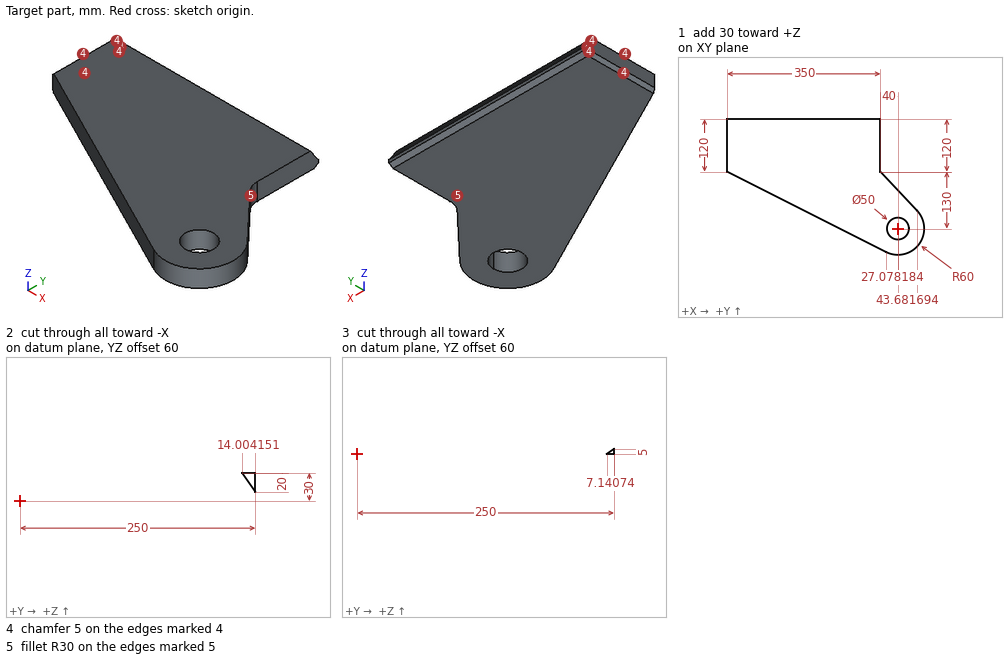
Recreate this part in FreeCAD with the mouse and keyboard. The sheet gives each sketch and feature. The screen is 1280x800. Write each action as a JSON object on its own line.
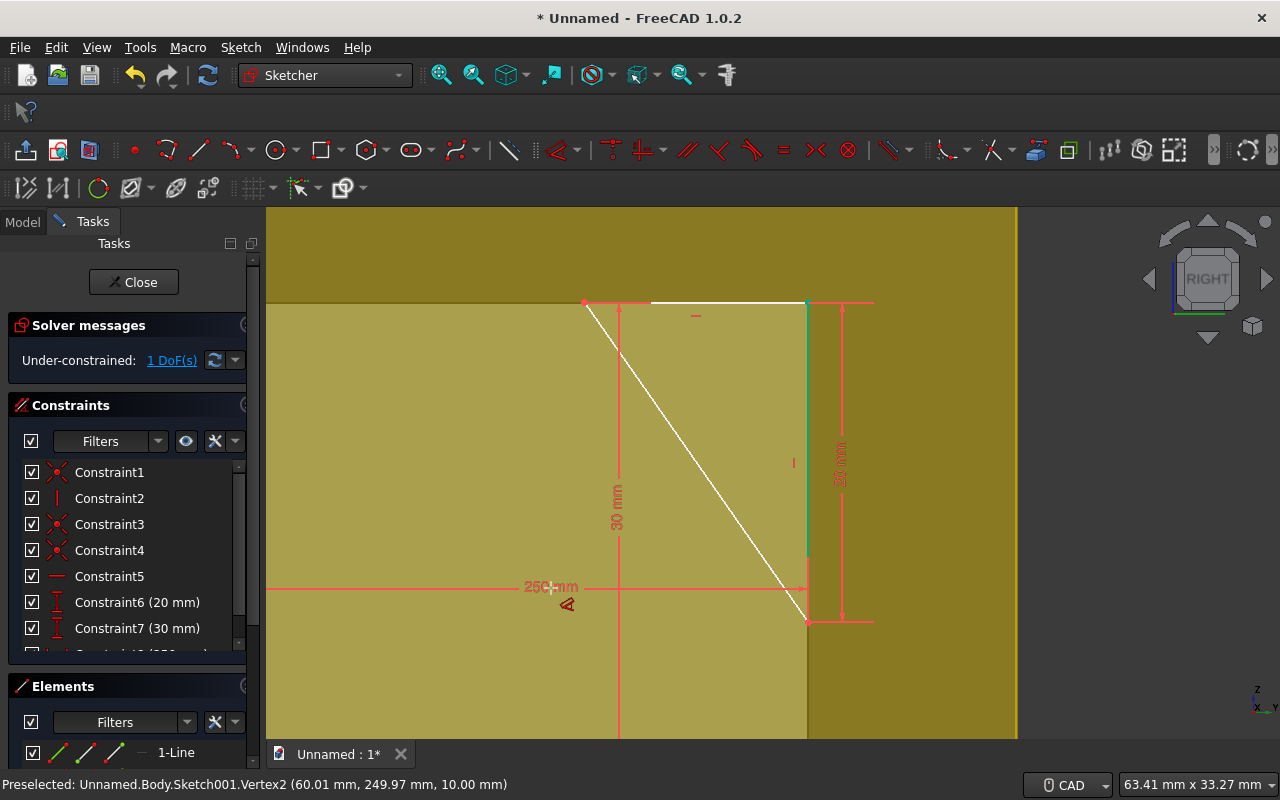
{"action": "left_click", "coordinate": [741, 303]}
{"action": "left_click", "coordinate": [696, 269]}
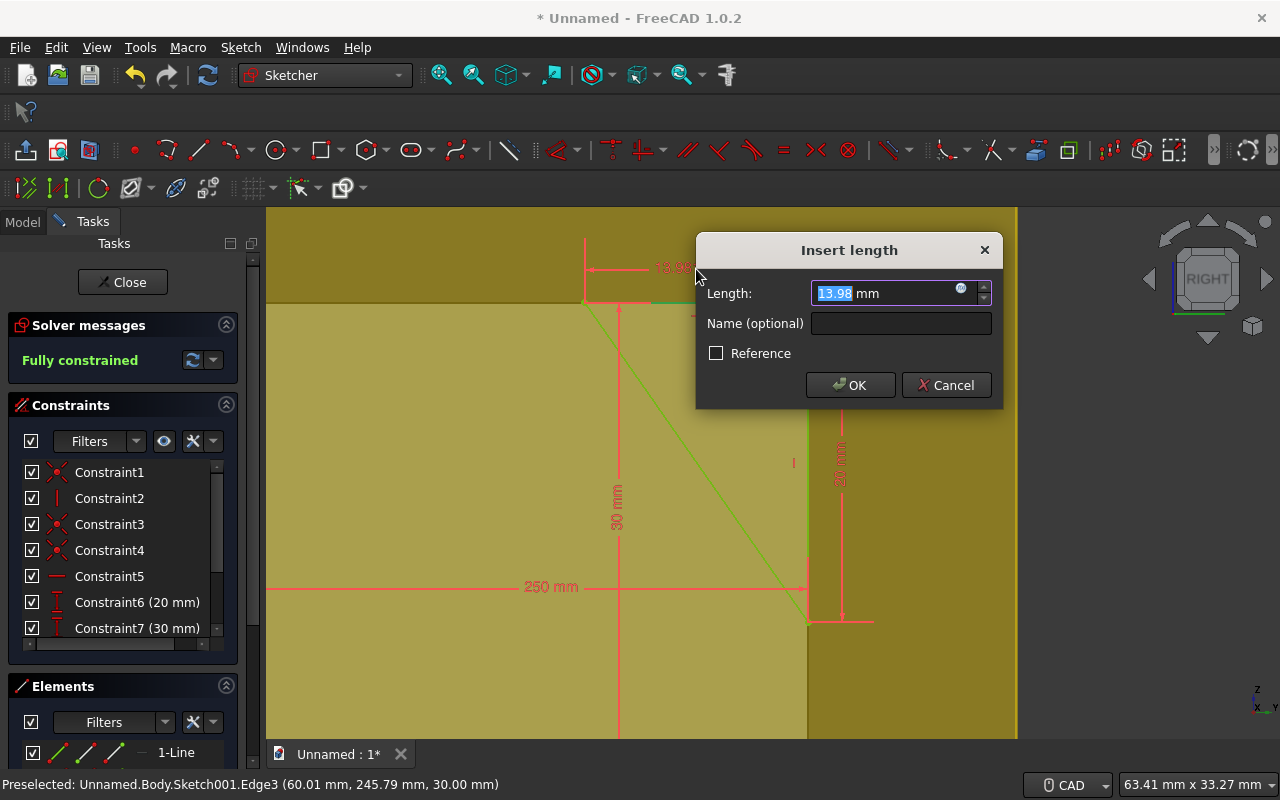
{"action": "type", "text": "14.004151"}
{"action": "key", "text": "Return"}
{"action": "key", "text": "Escape"}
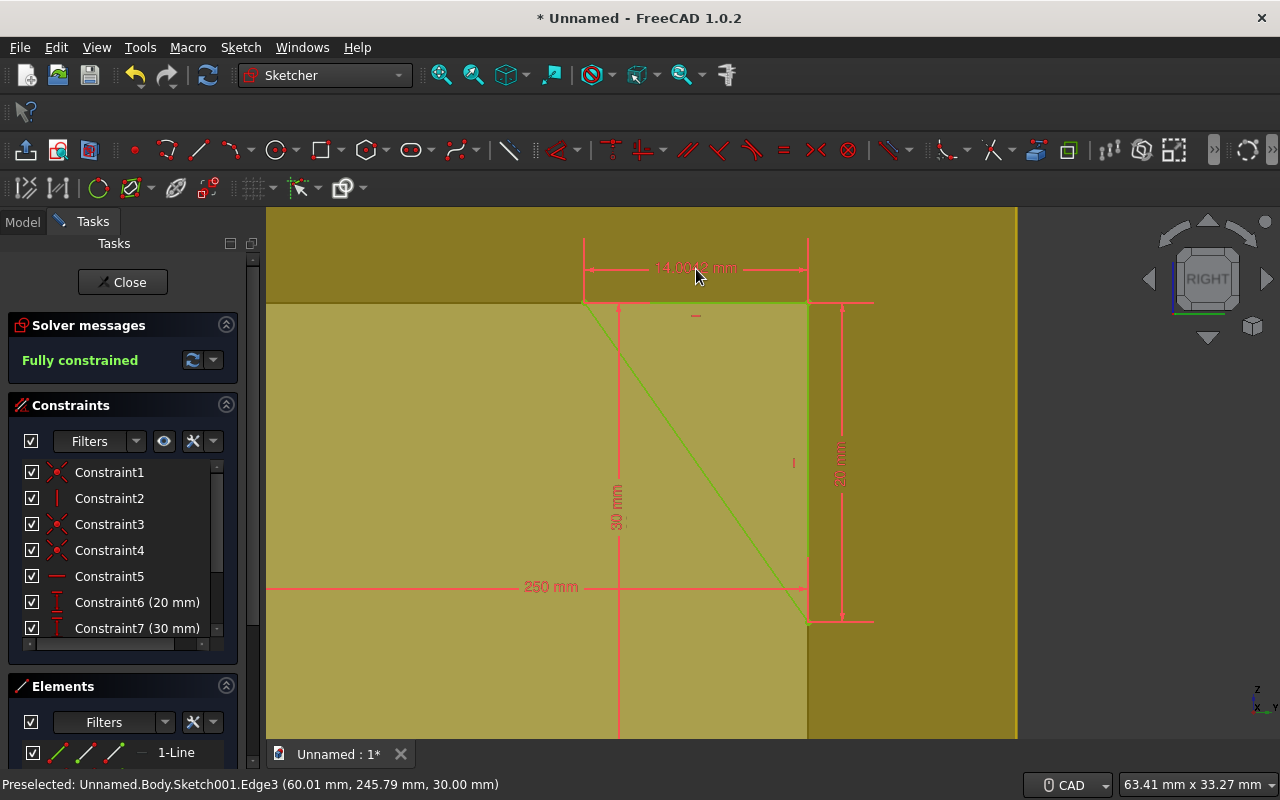
{"action": "left_click", "coordinate": [123, 282]}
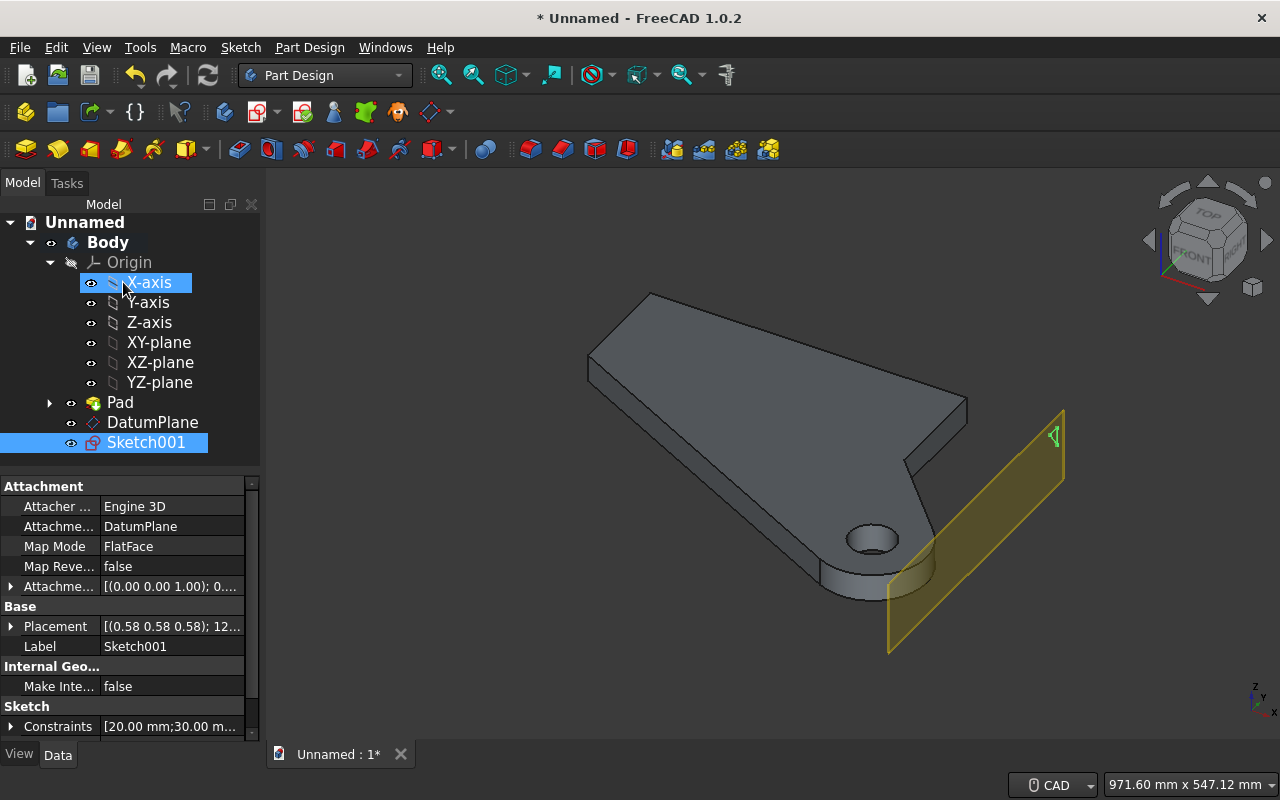
{"action": "left_click", "coordinate": [240, 150]}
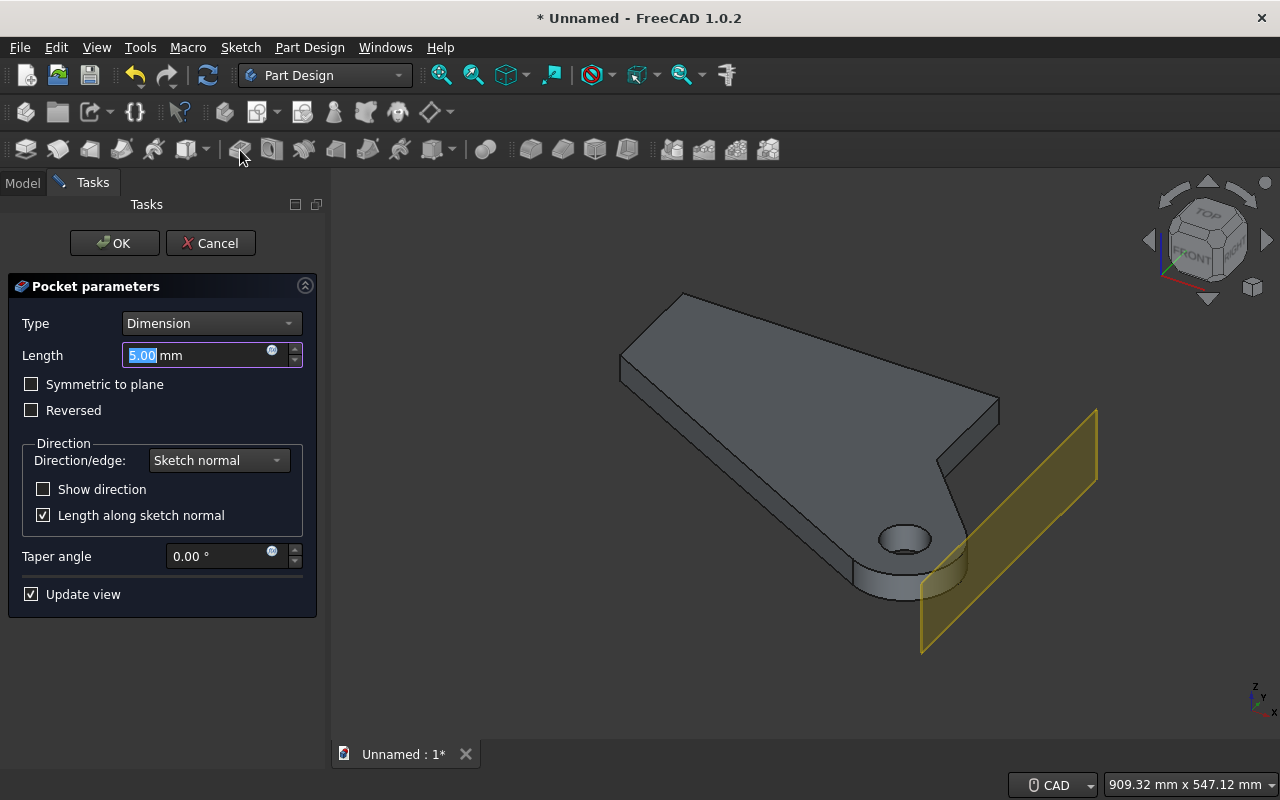
{"action": "left_click", "coordinate": [212, 324]}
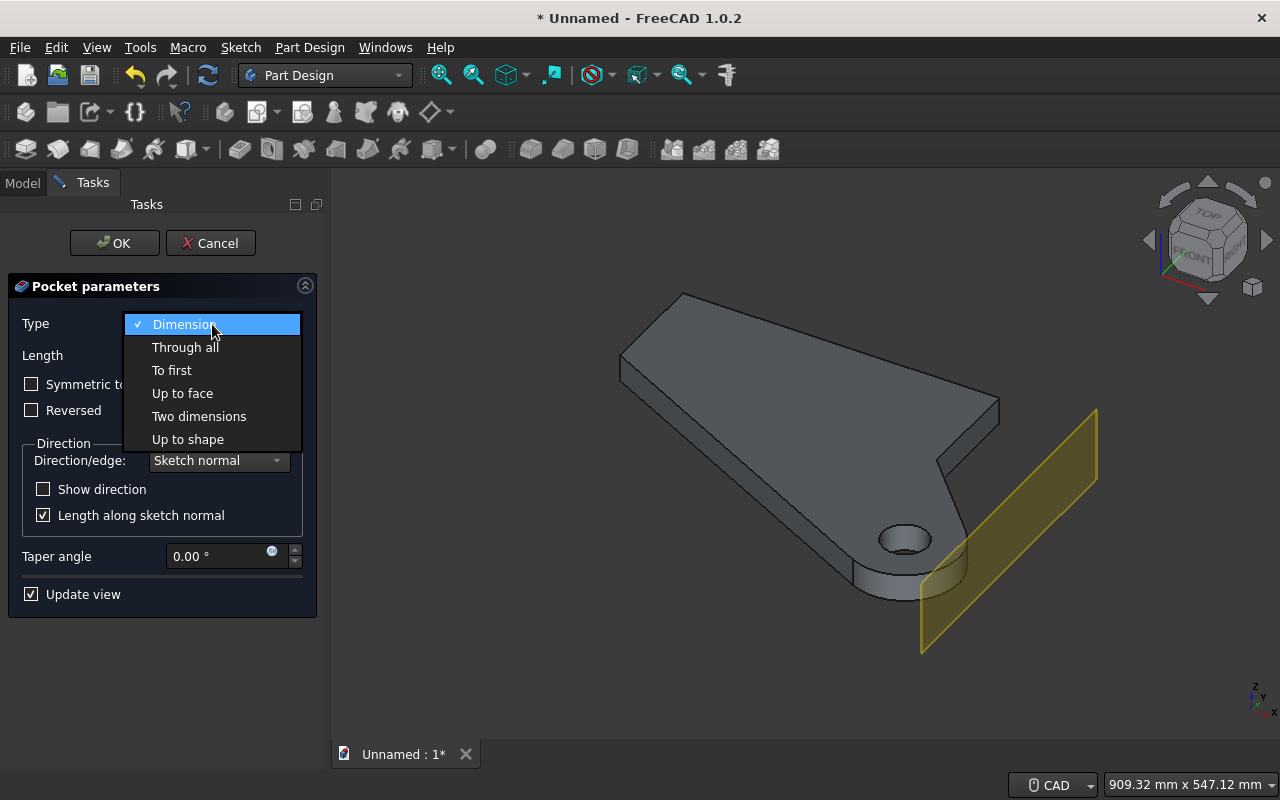
{"action": "left_click", "coordinate": [212, 348]}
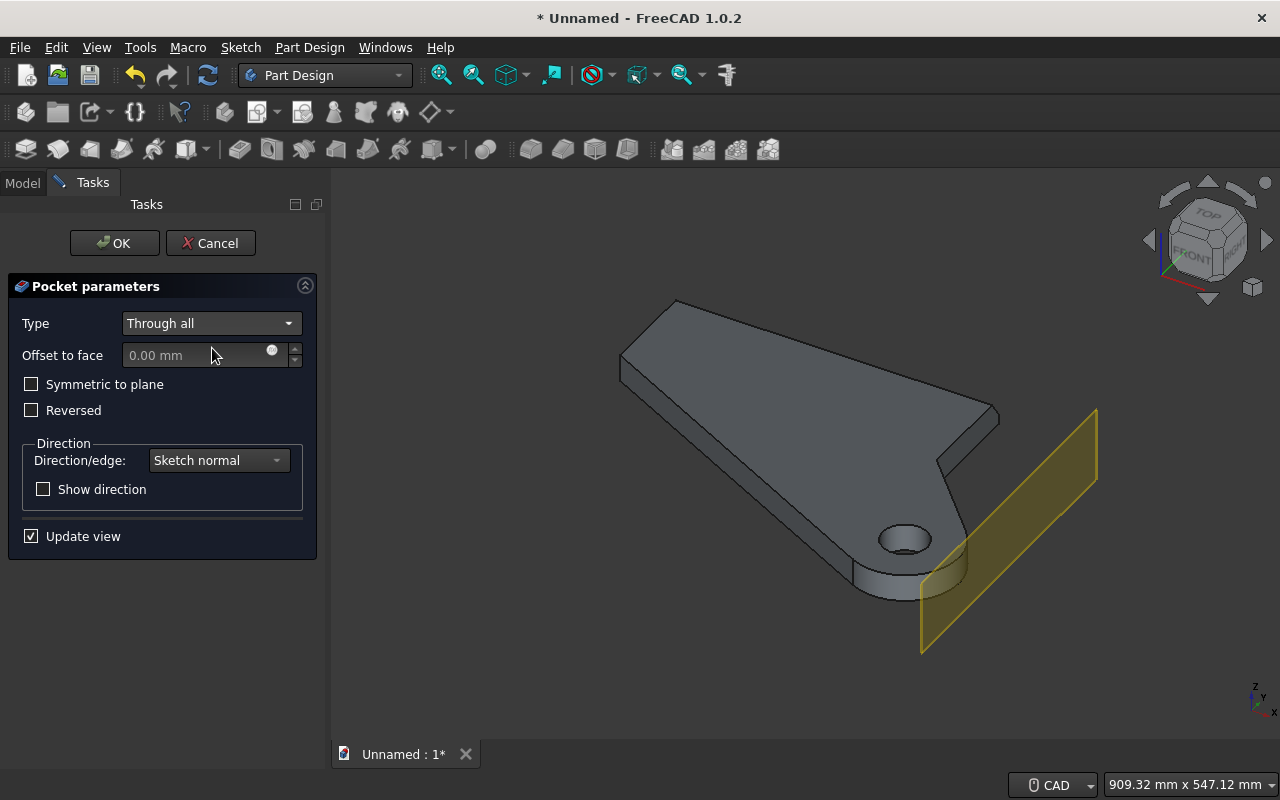
{"action": "left_click", "coordinate": [115, 243]}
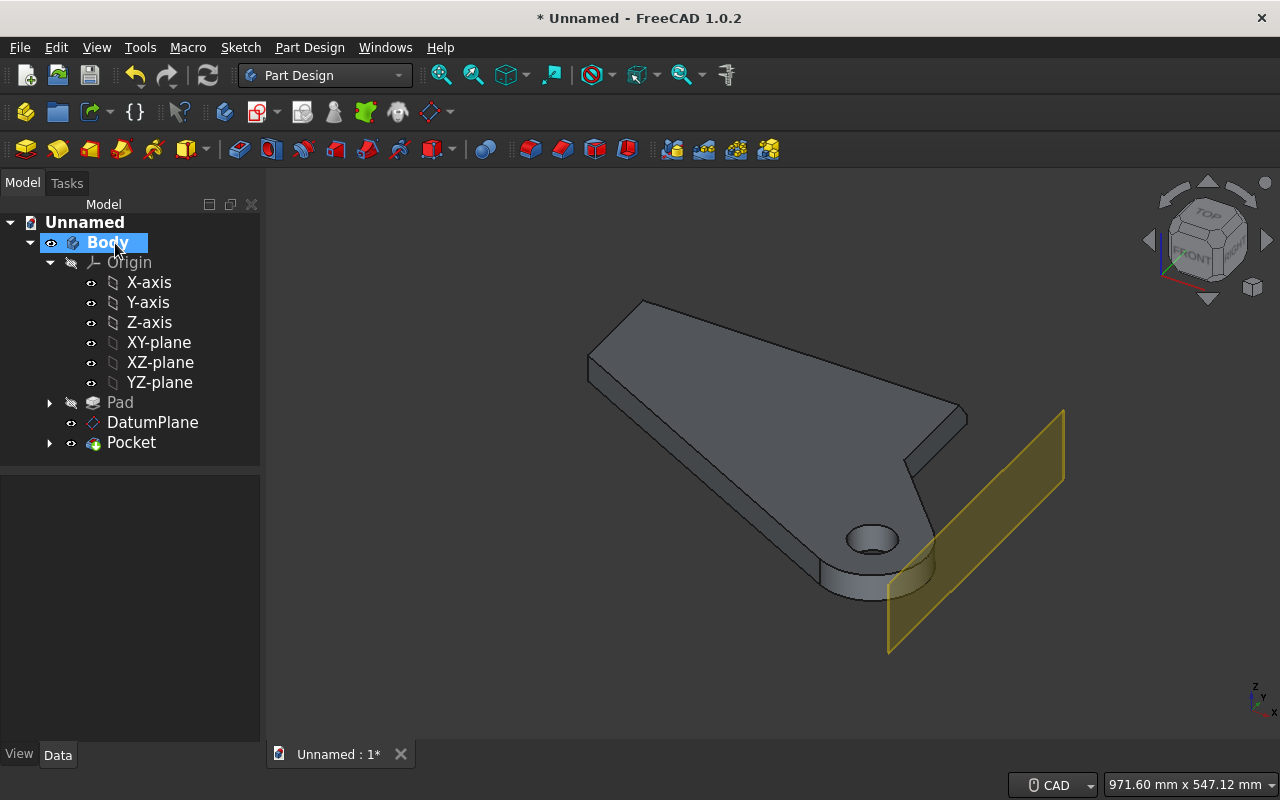
{"action": "left_click", "coordinate": [116, 423]}
{"action": "key", "text": "space"}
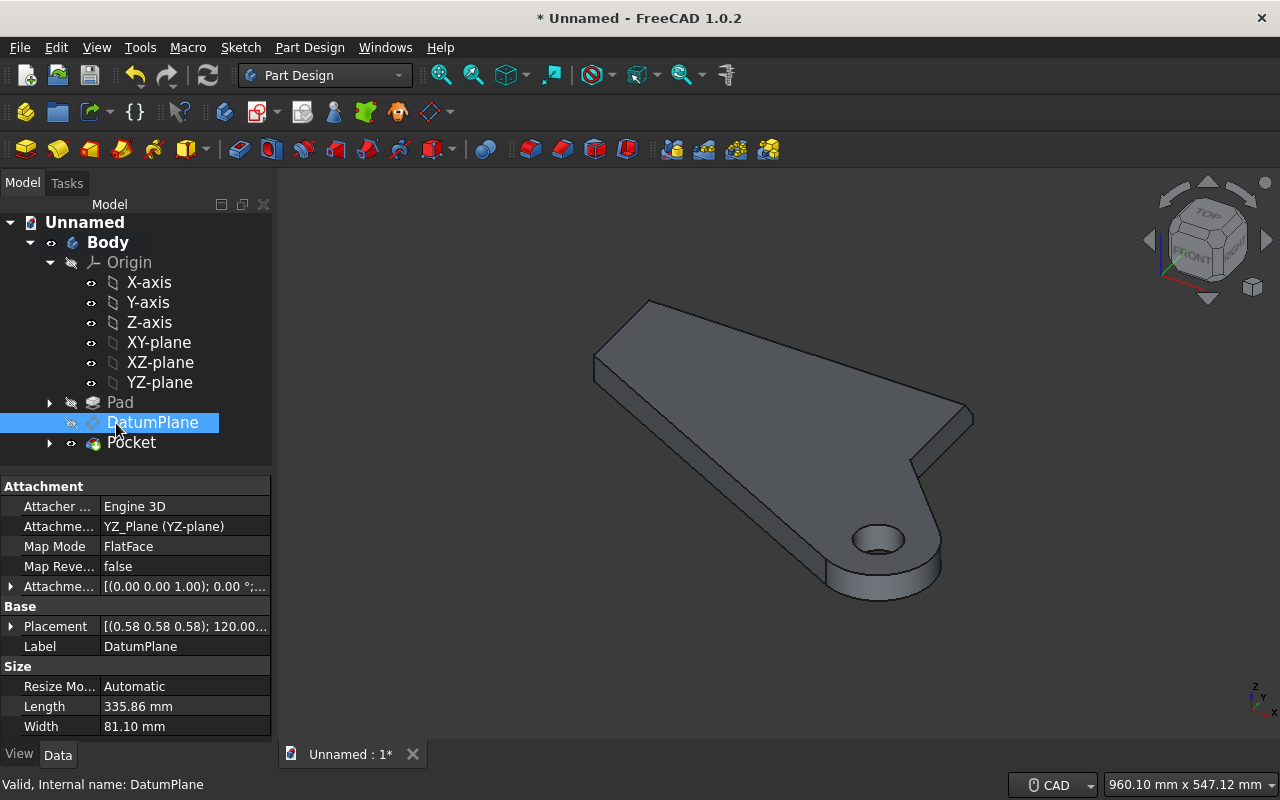
{"action": "left_click", "coordinate": [136, 383]}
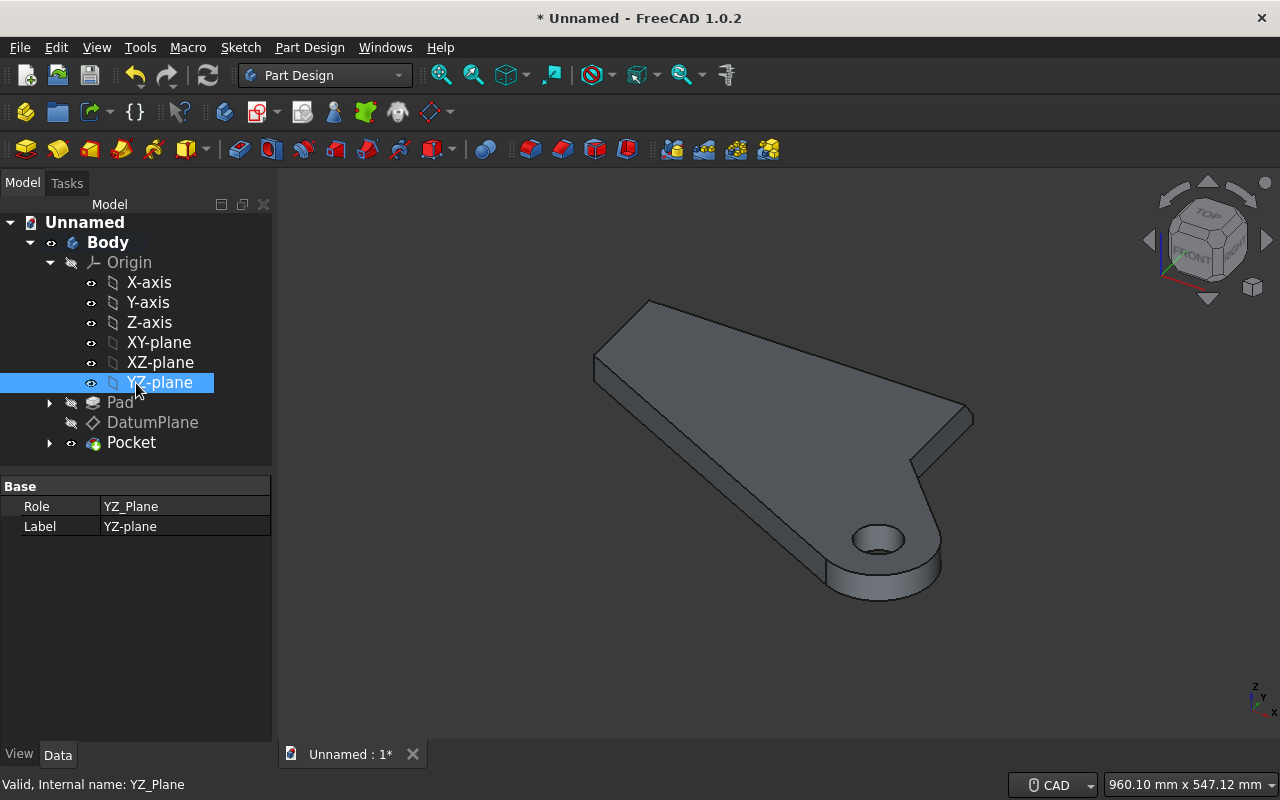
{"action": "left_click", "coordinate": [430, 112]}